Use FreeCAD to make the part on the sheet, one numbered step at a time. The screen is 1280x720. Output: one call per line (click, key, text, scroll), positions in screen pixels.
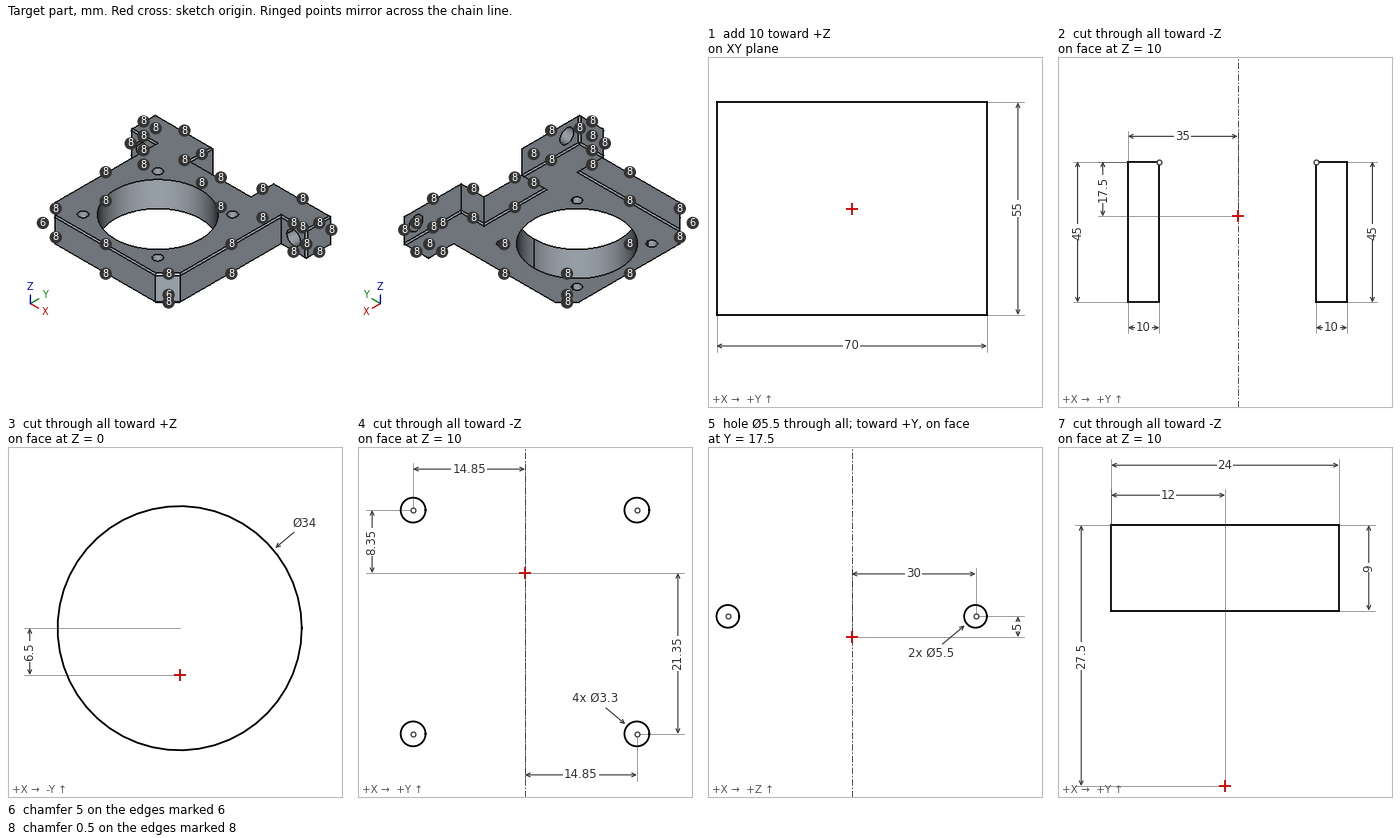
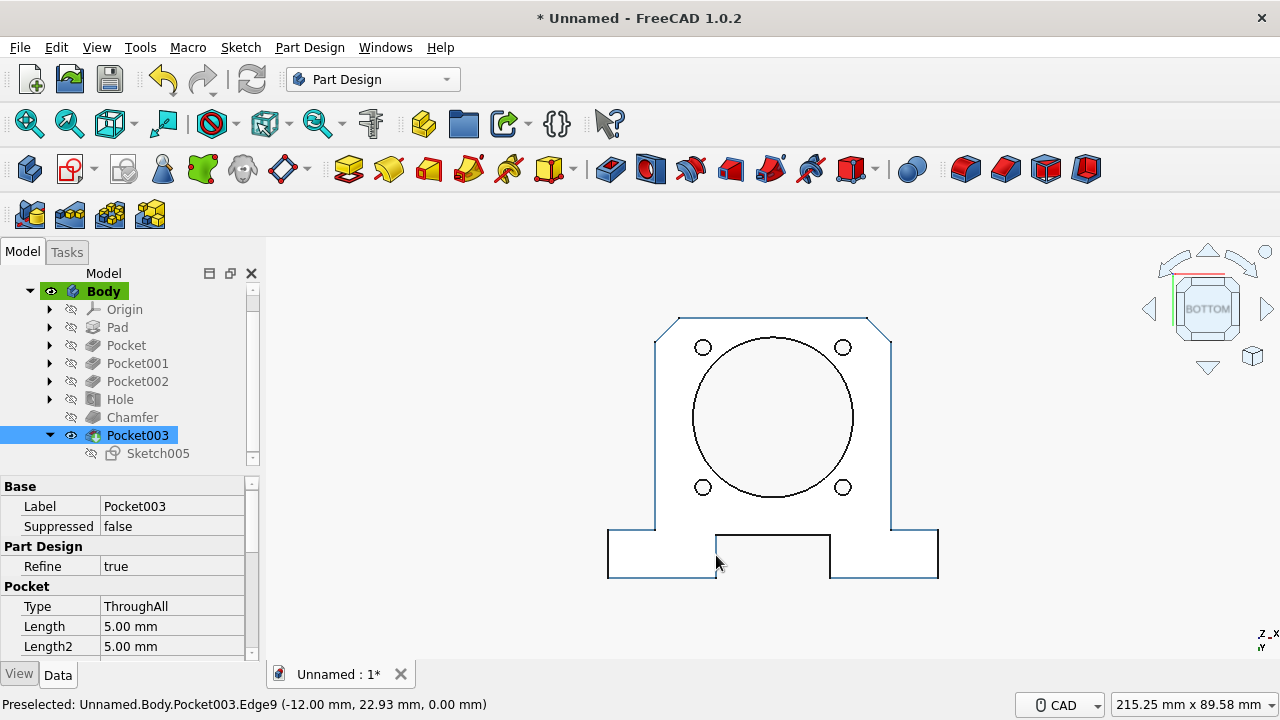
click(830, 555, ctrl)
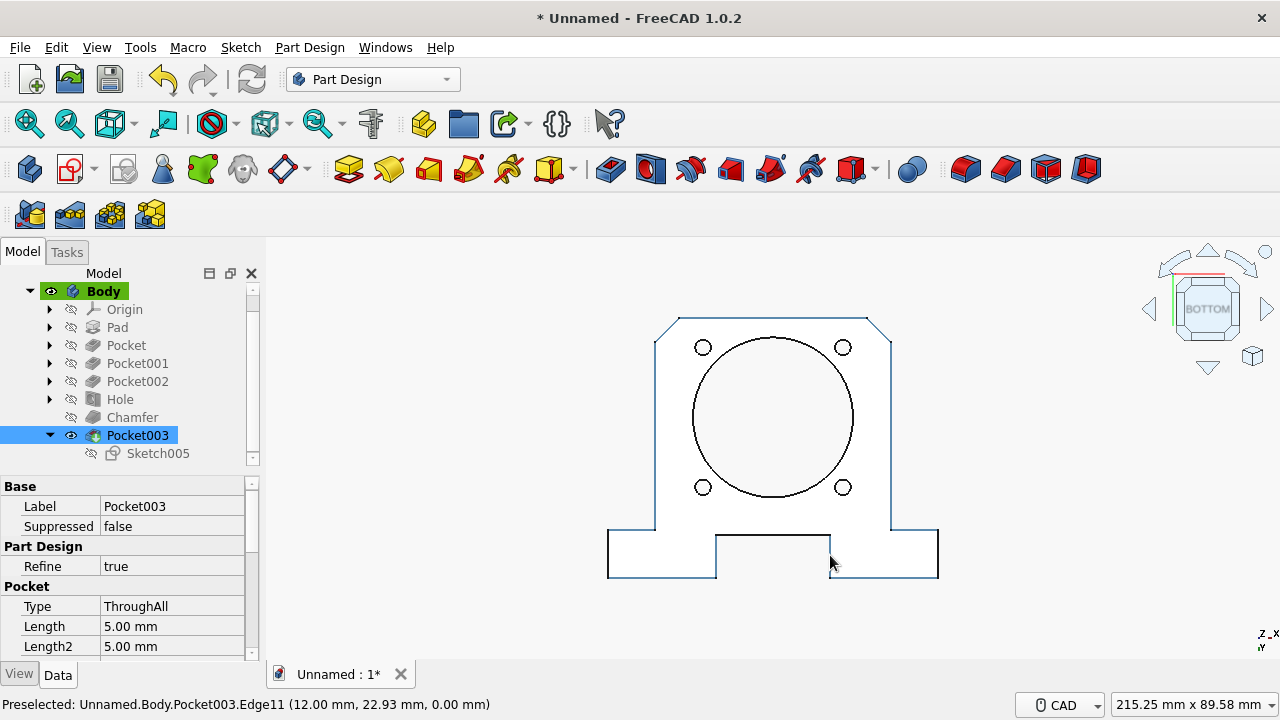
click(773, 534, ctrl)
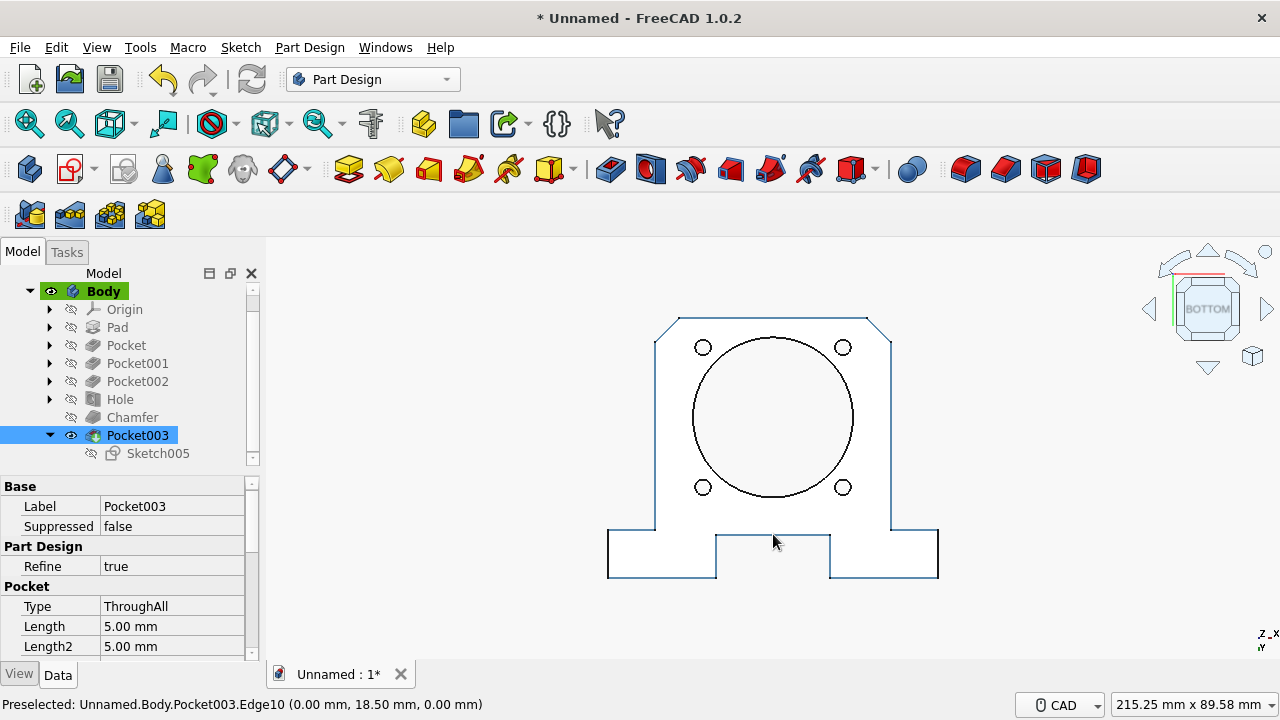
key(4)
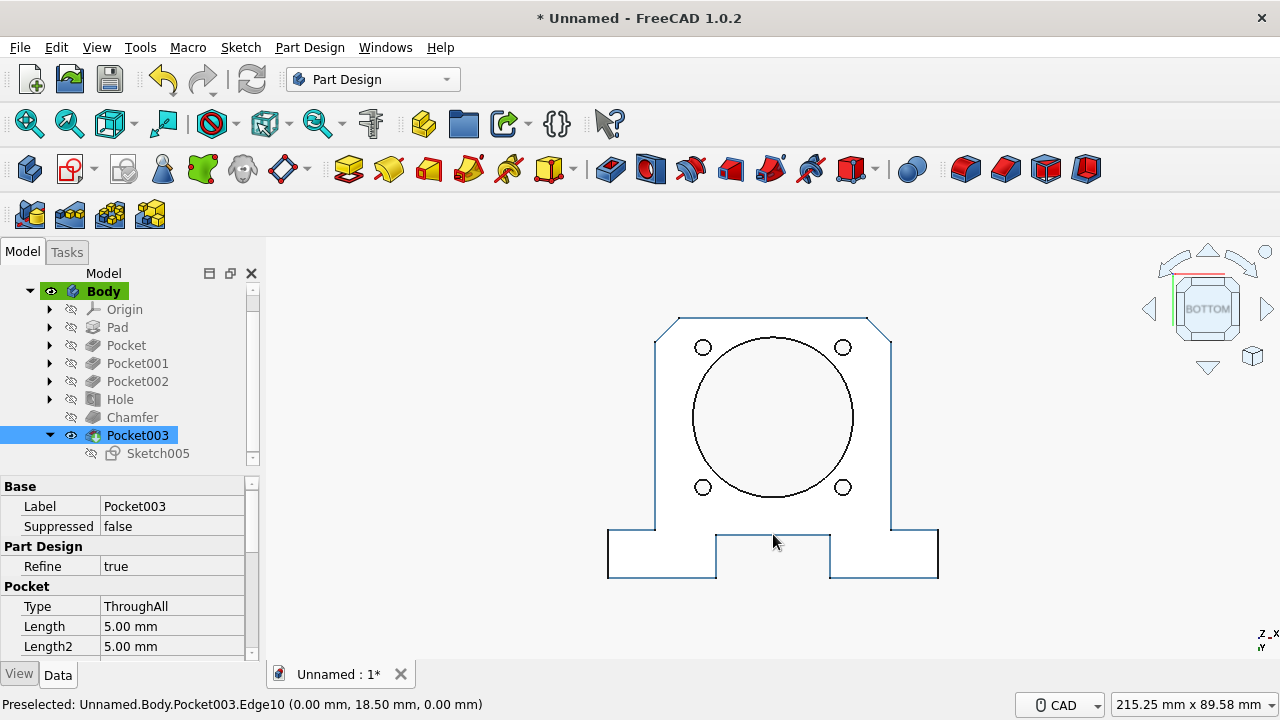
click(30, 124)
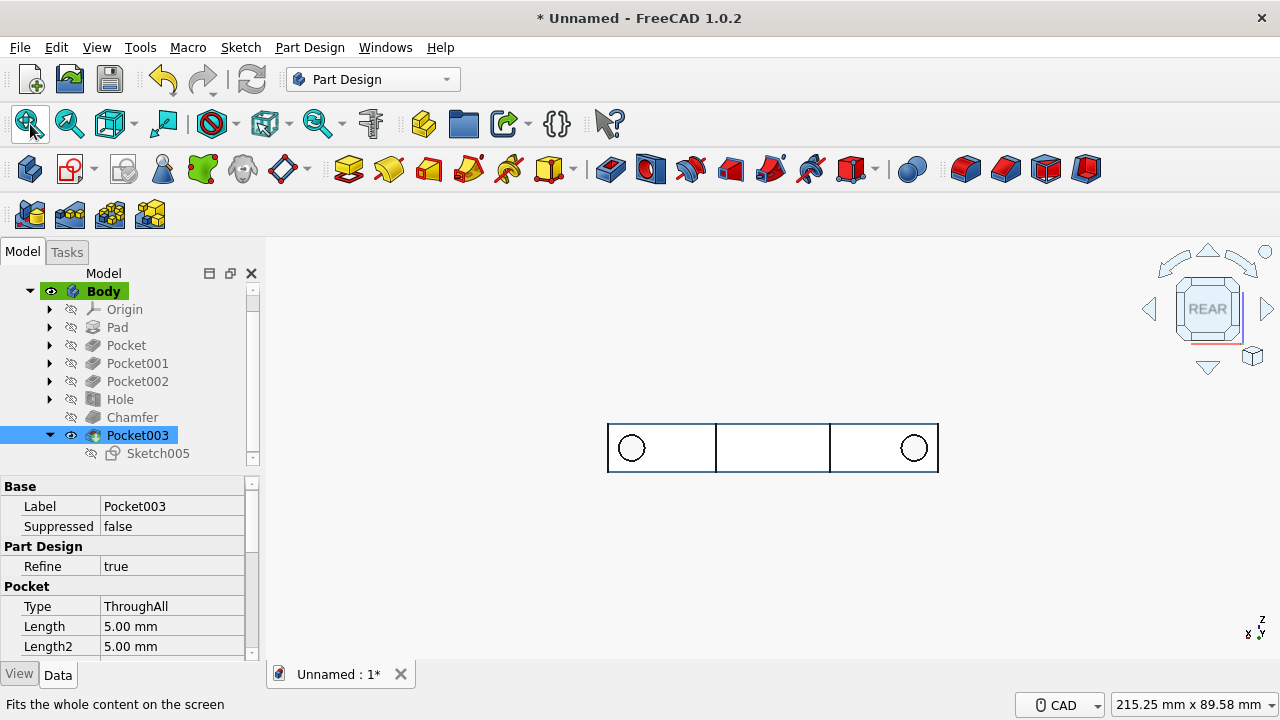
key(6)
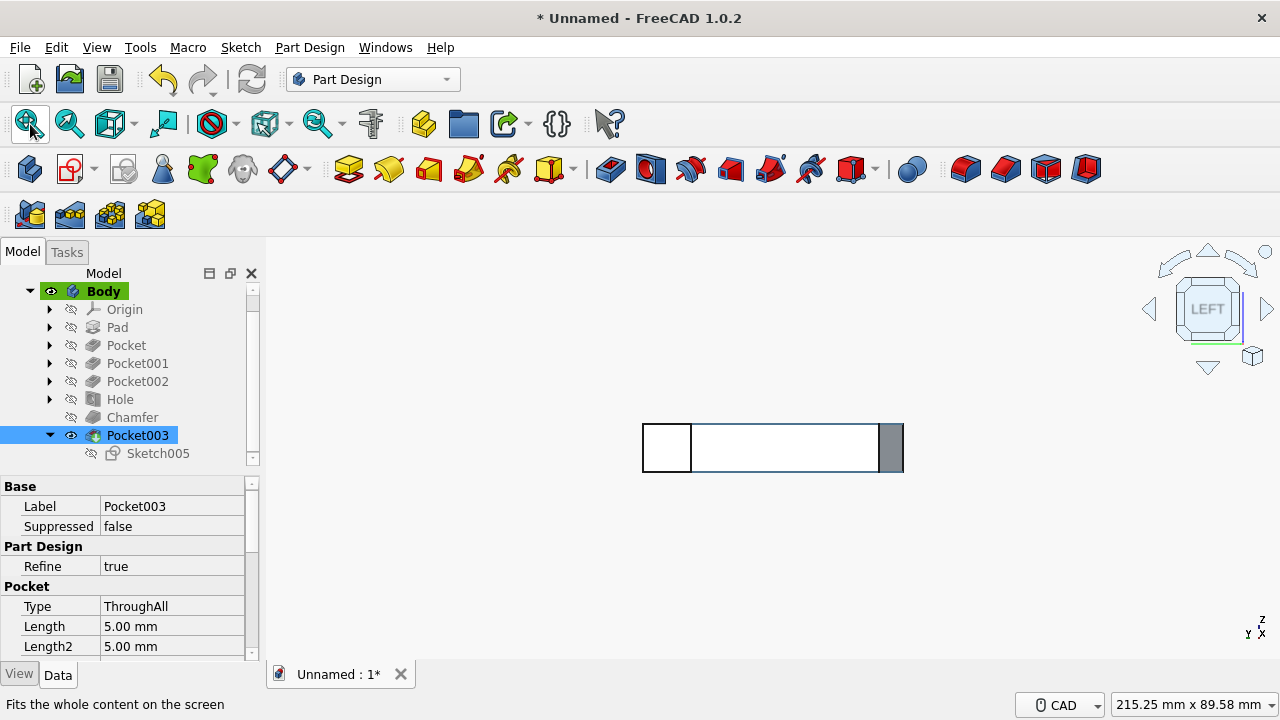
key(v)
key(f)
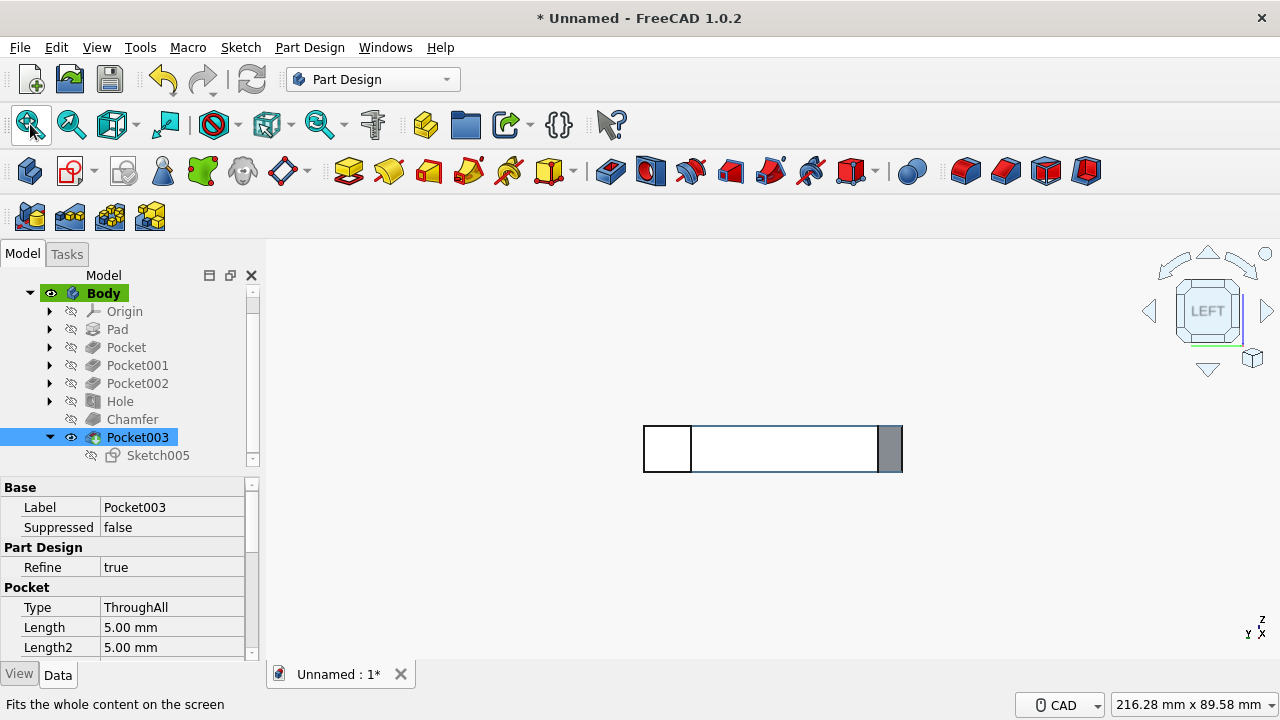
click(668, 448, ctrl)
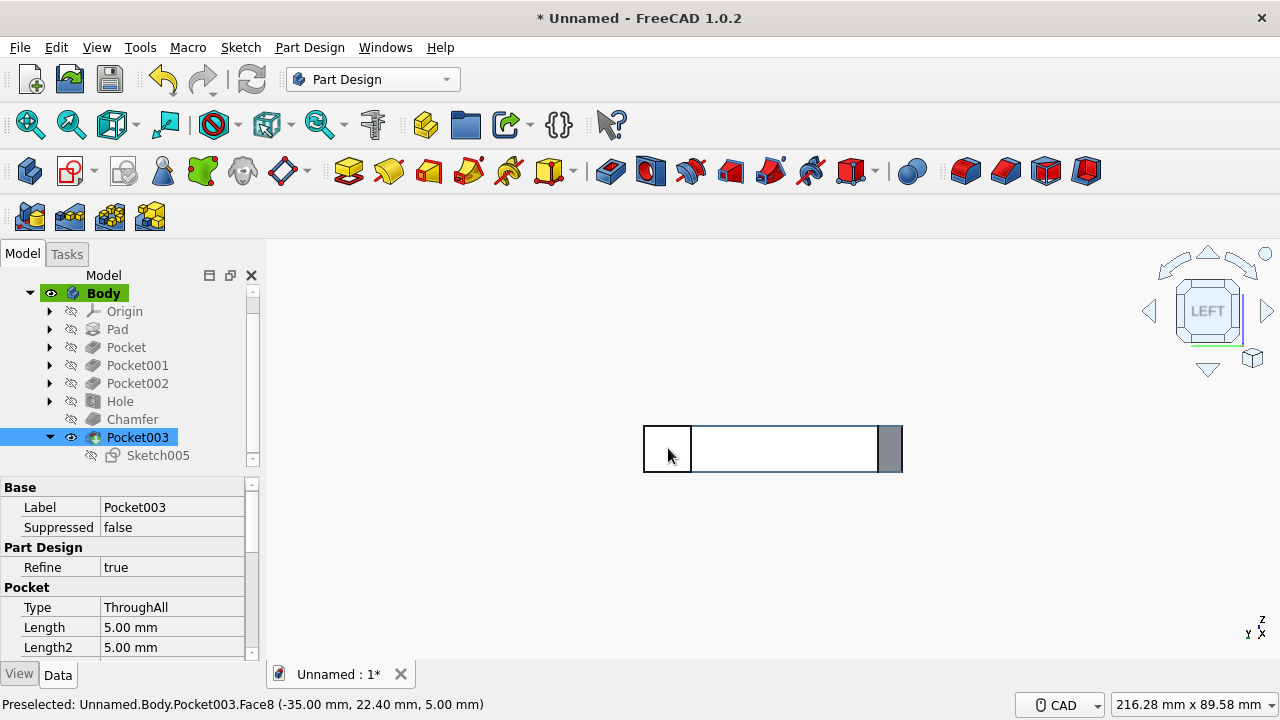
click(1006, 172)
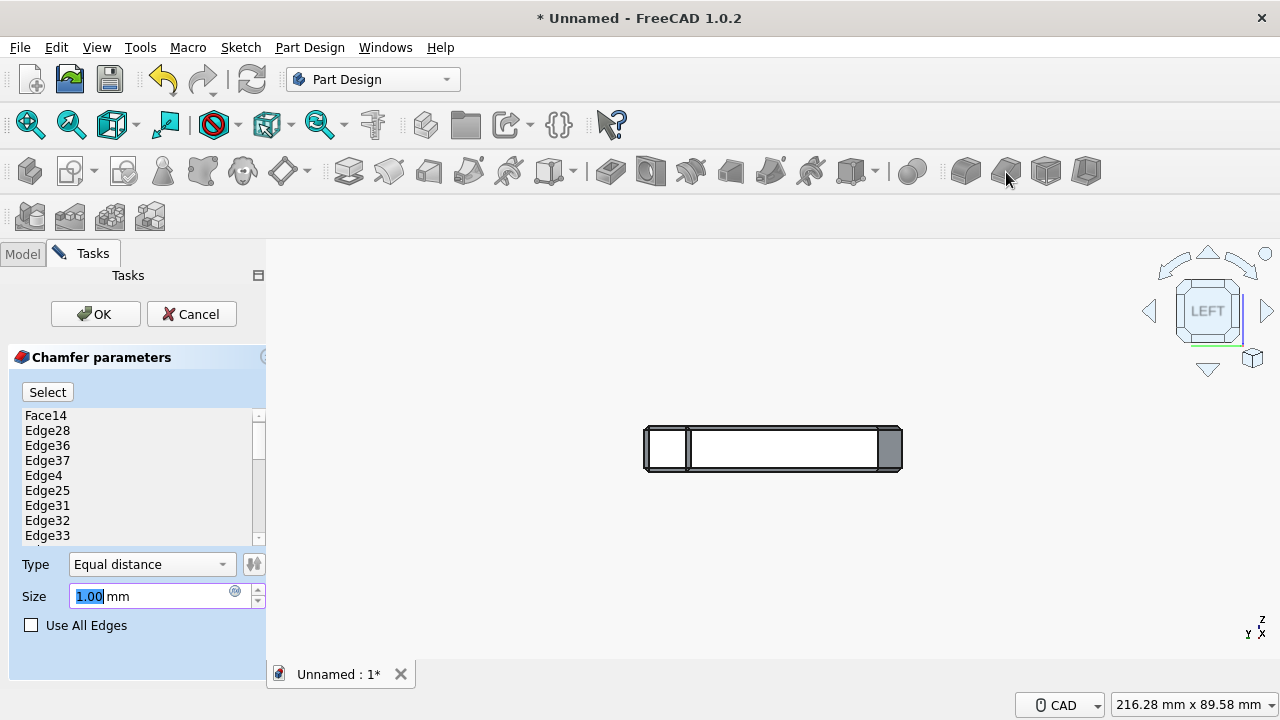
text(0.5)
key(Tab)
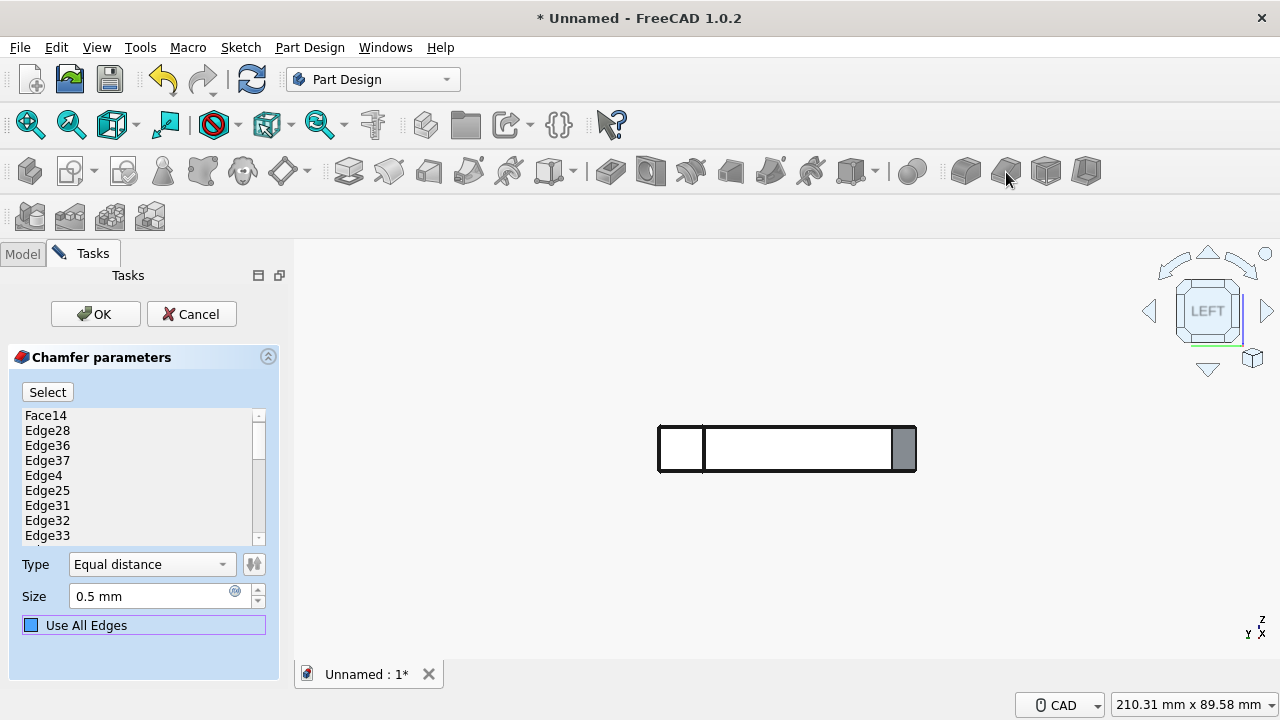
click(96, 314)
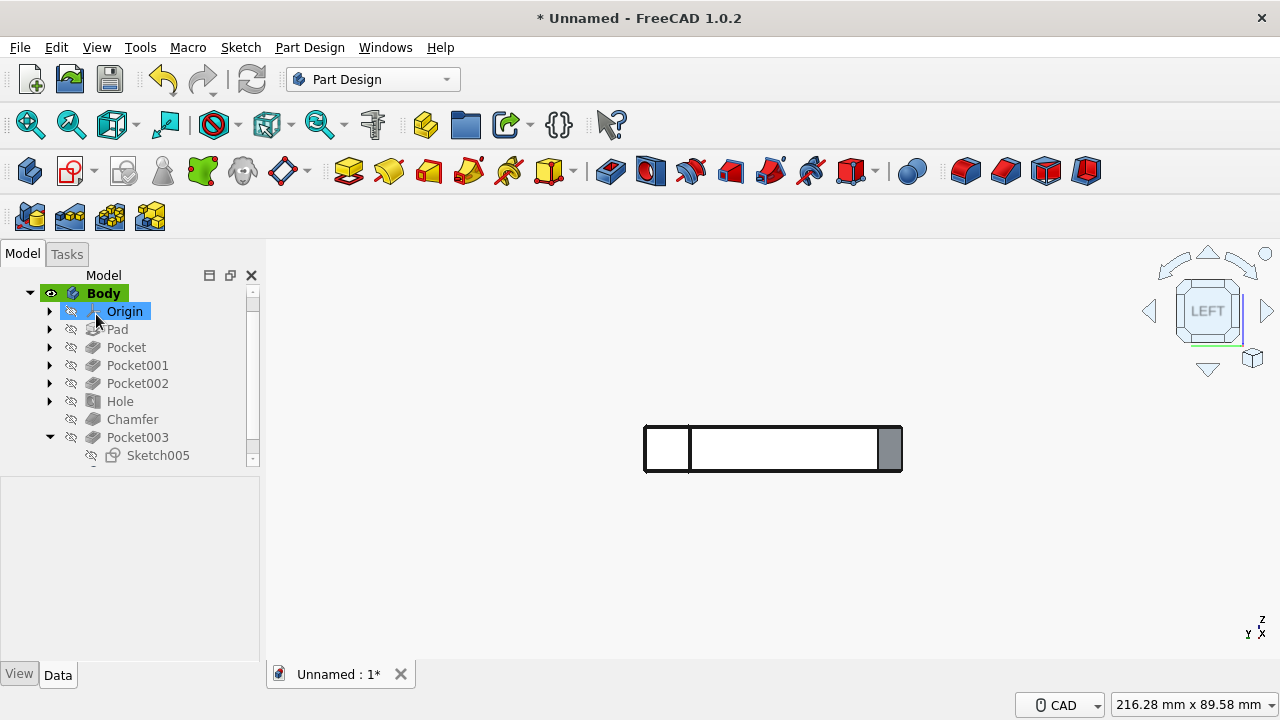
key(0)